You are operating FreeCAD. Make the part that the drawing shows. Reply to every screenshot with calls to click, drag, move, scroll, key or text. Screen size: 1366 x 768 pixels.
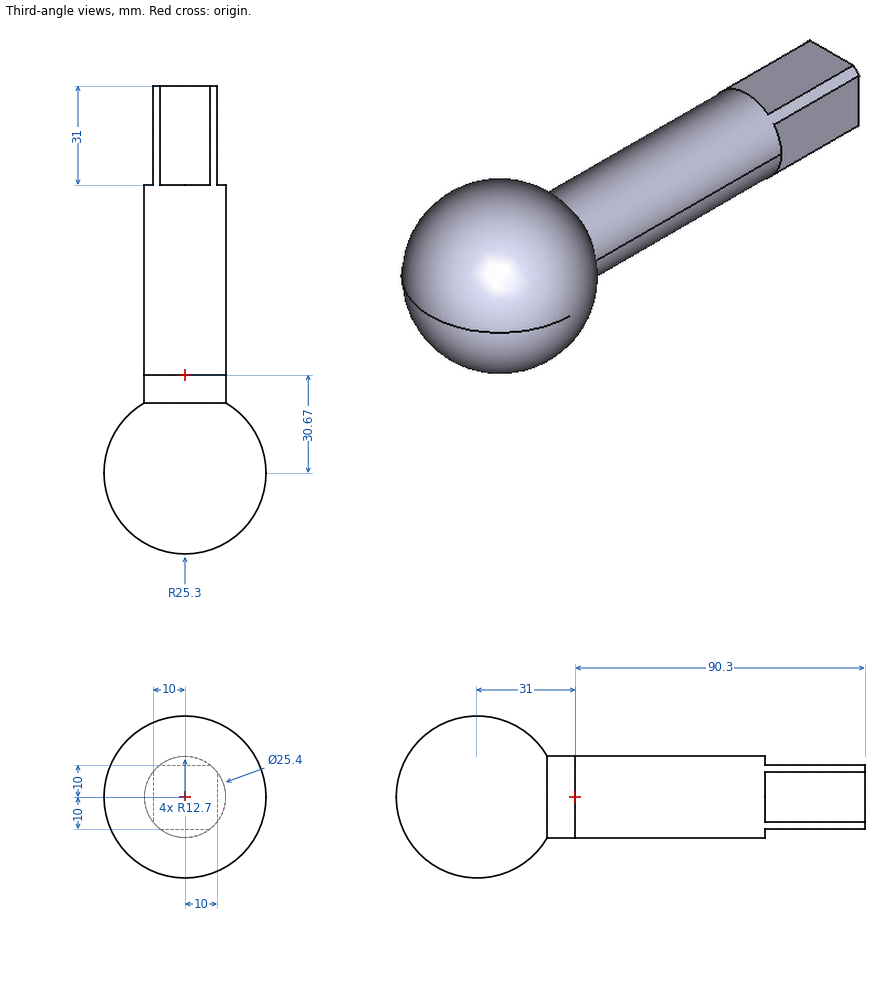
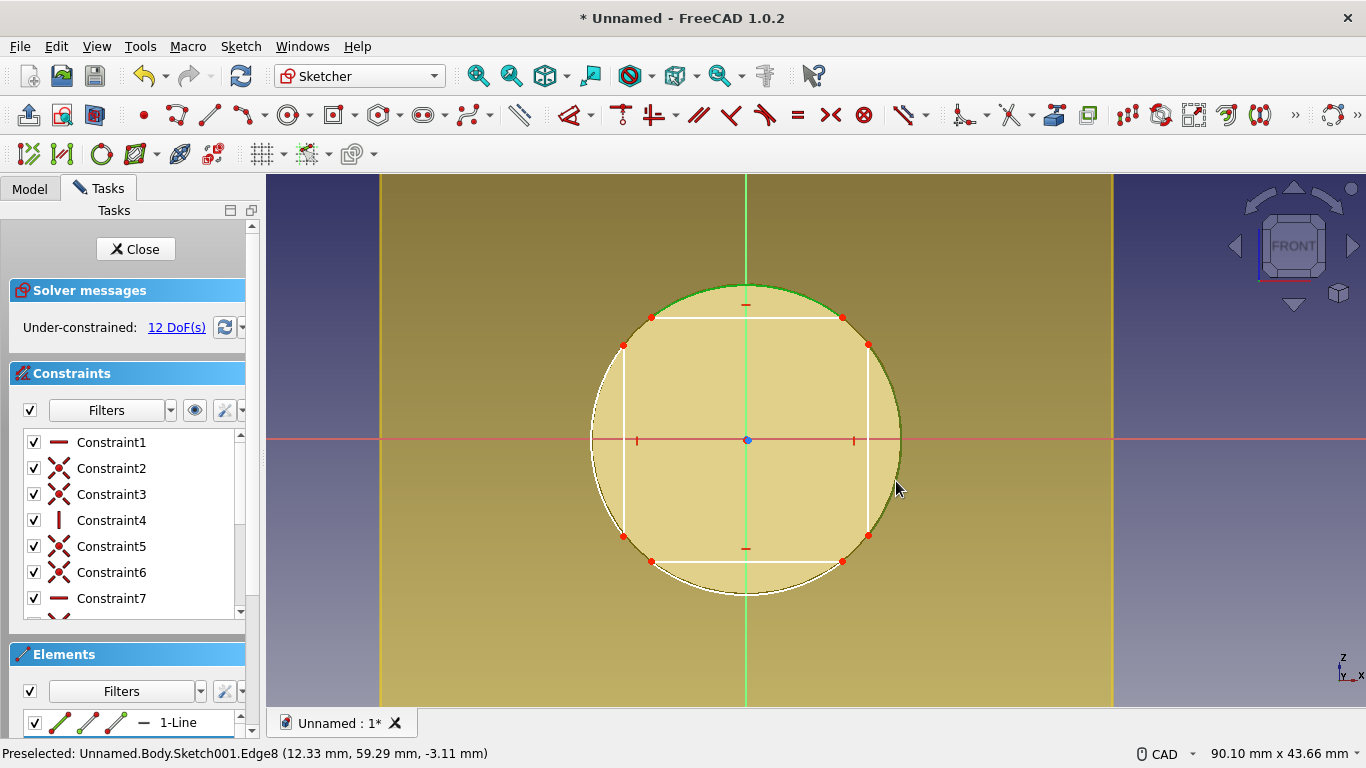
click(621, 116)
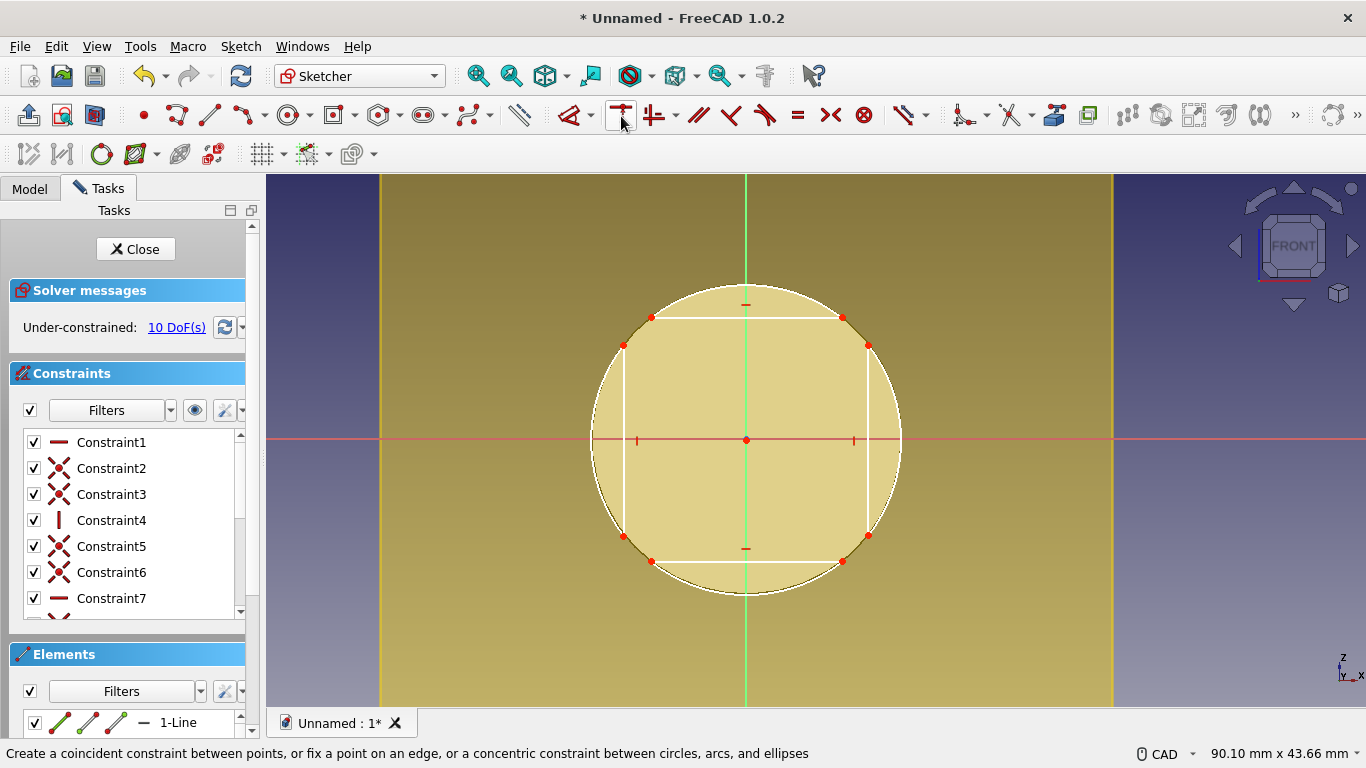
drag(736, 429, 756, 451)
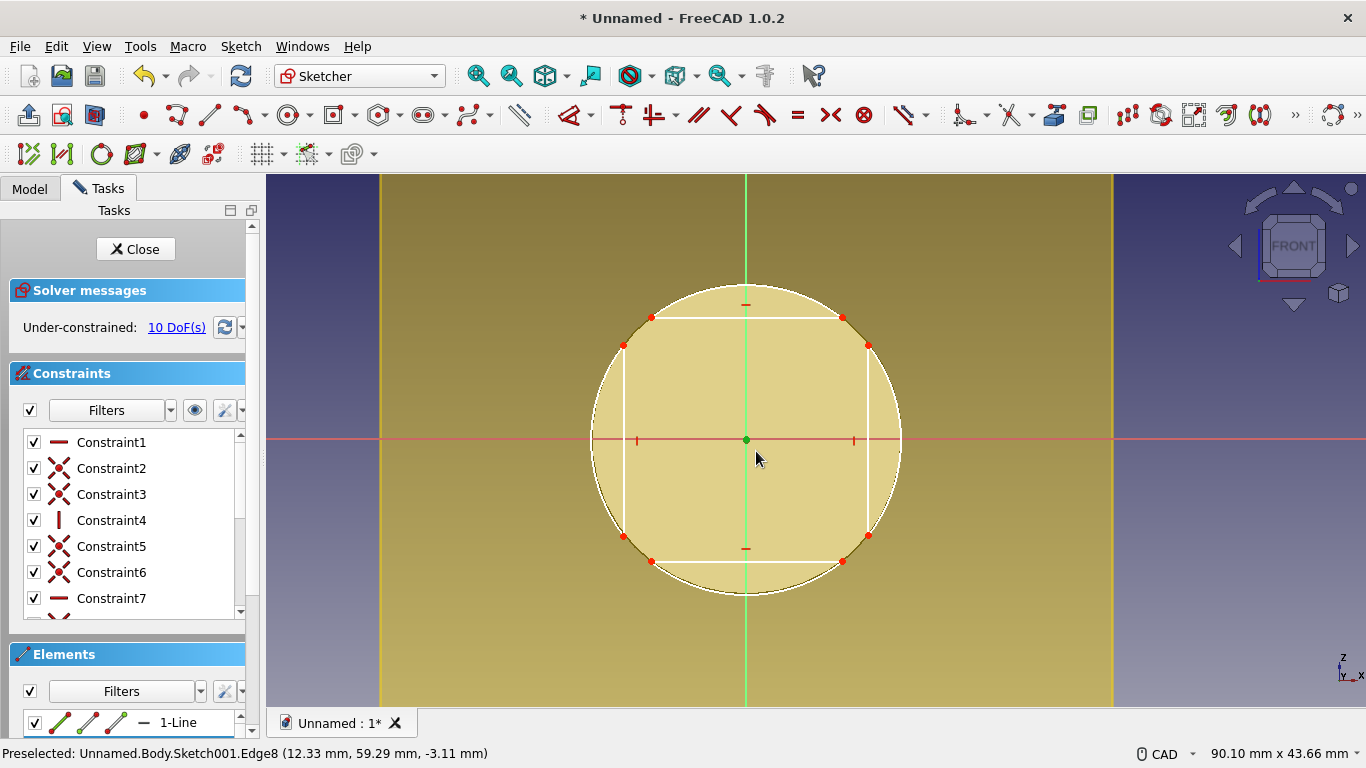
click(621, 116)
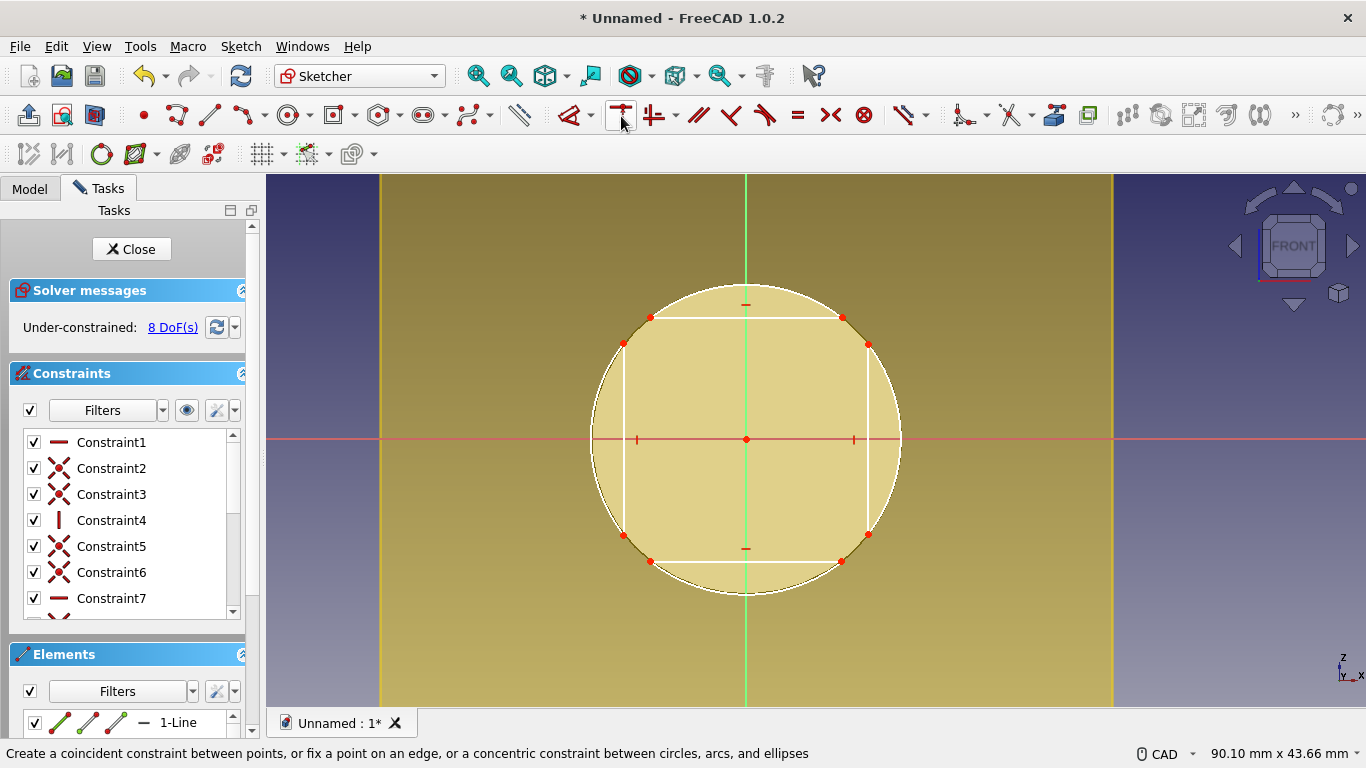
click(787, 290)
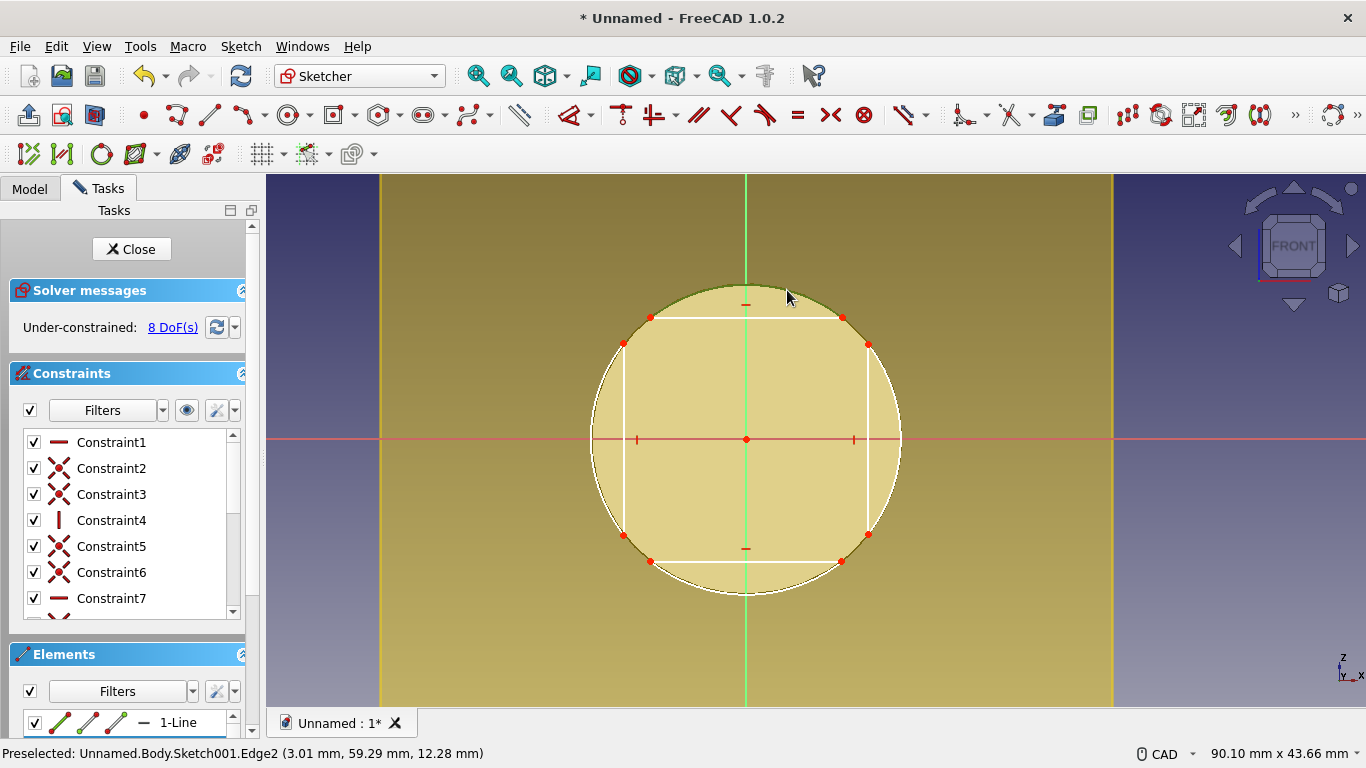
click(596, 398)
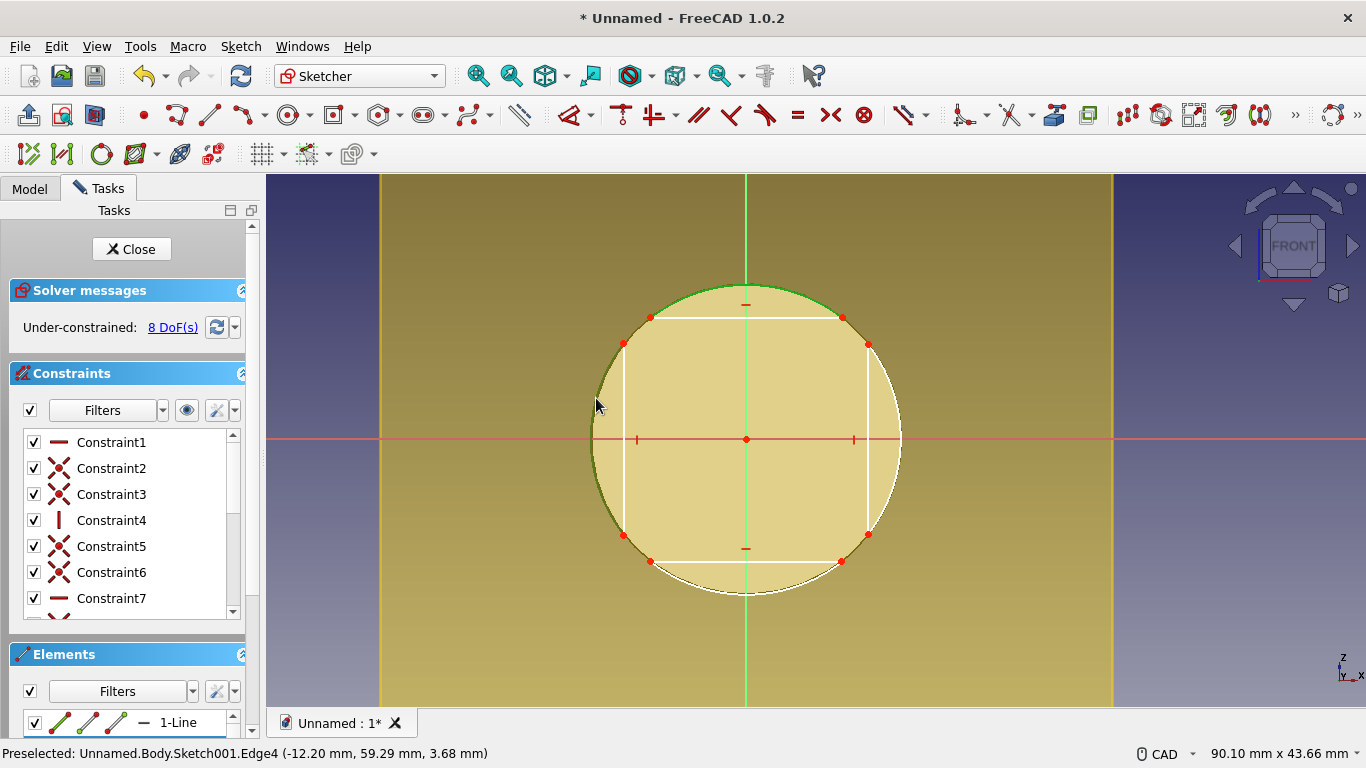
click(706, 589)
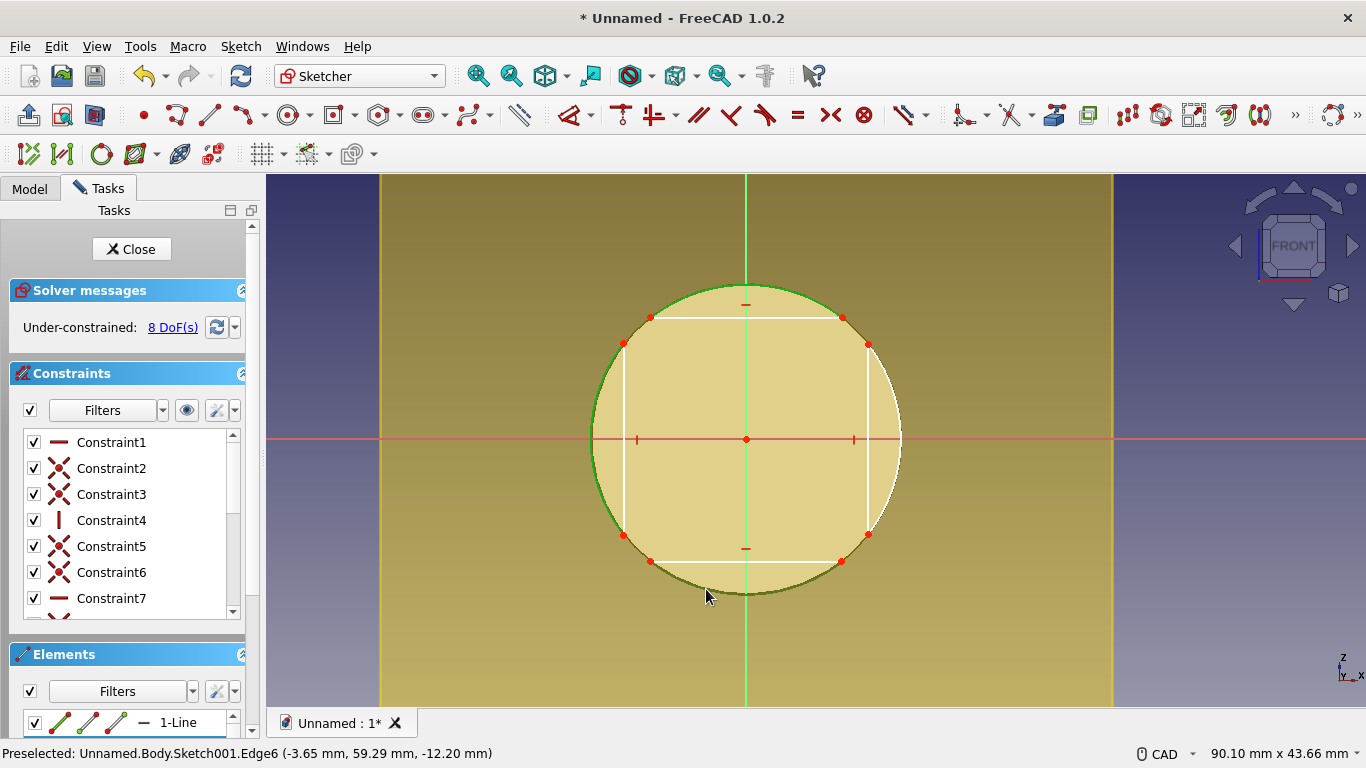
click(895, 480)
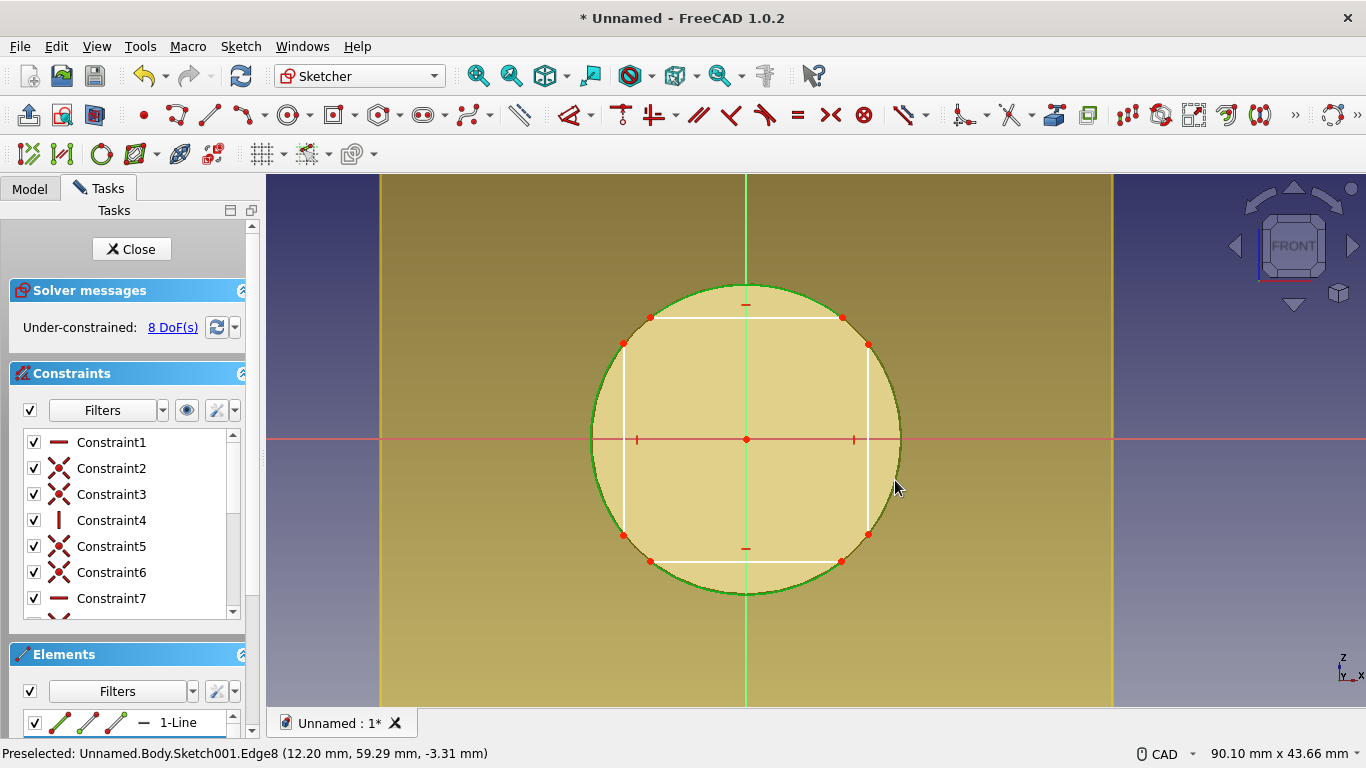
click(798, 116)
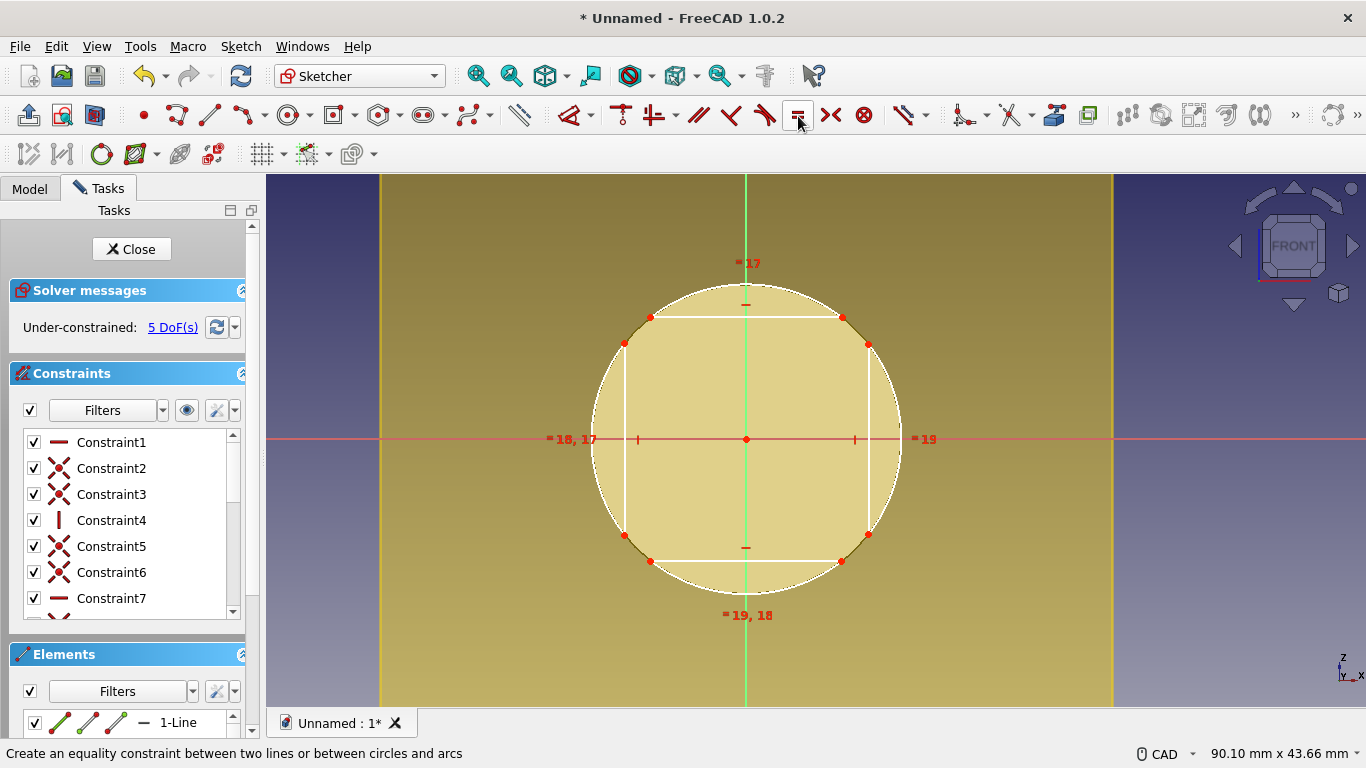
click(568, 116)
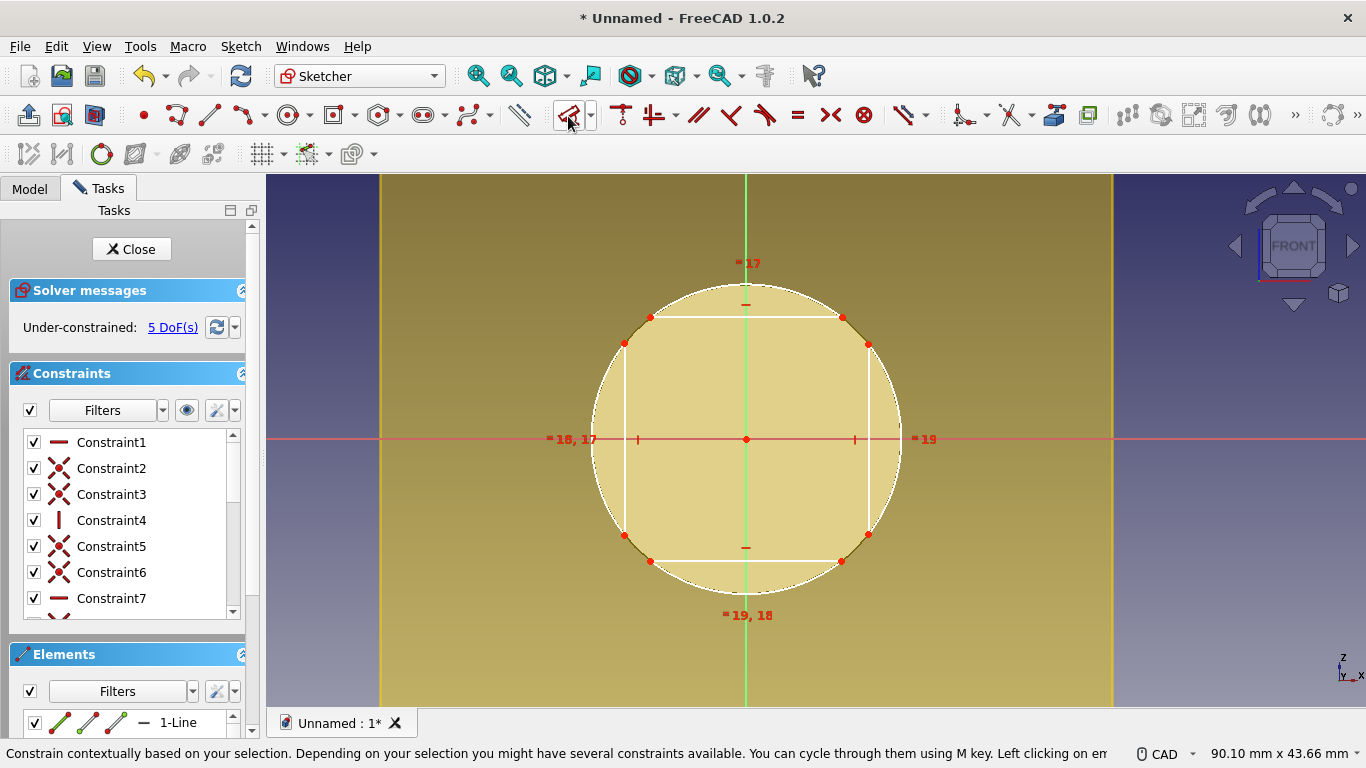
click(787, 290)
click(795, 259)